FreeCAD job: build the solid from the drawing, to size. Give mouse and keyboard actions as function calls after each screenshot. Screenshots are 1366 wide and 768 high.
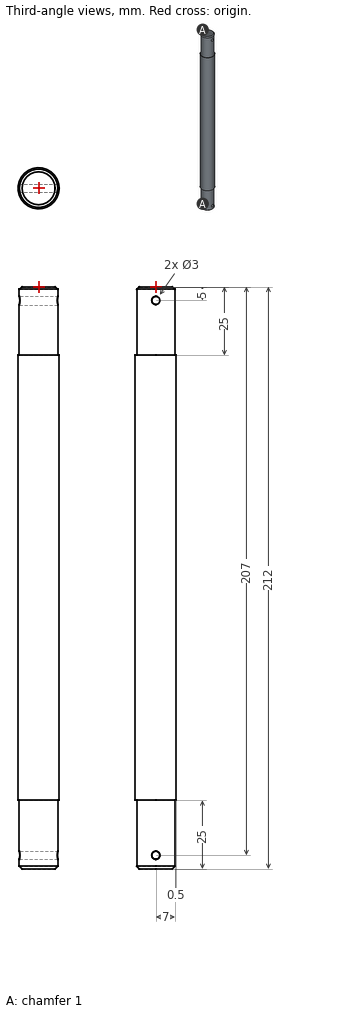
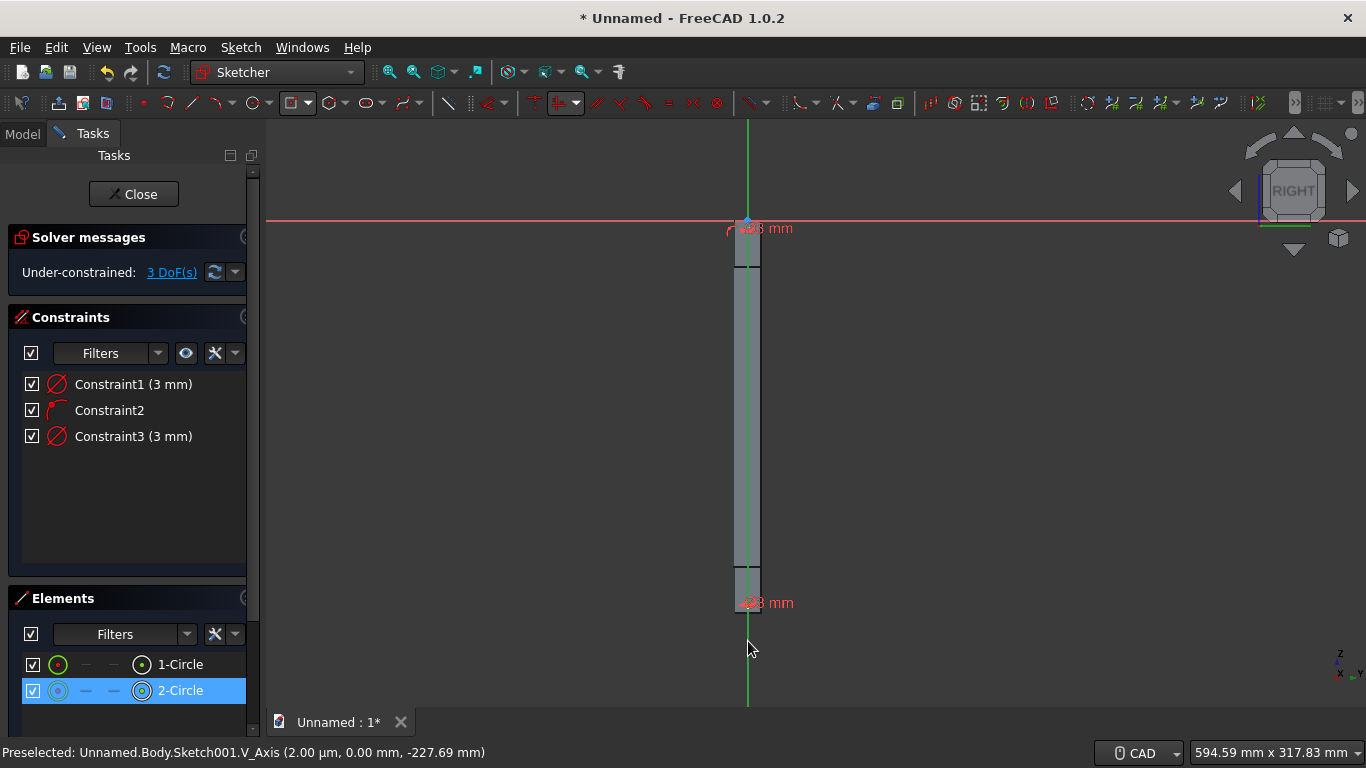
key(c)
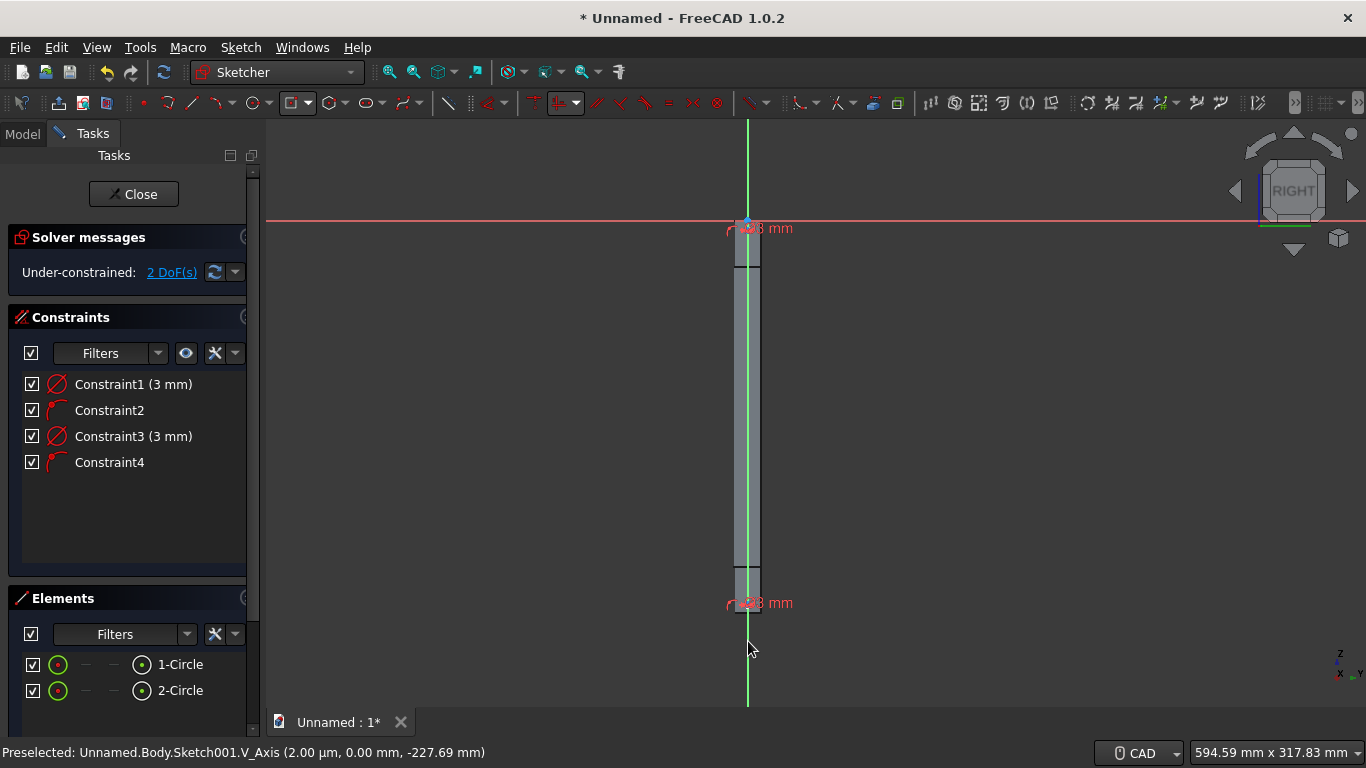
scroll(748, 230, up, 8)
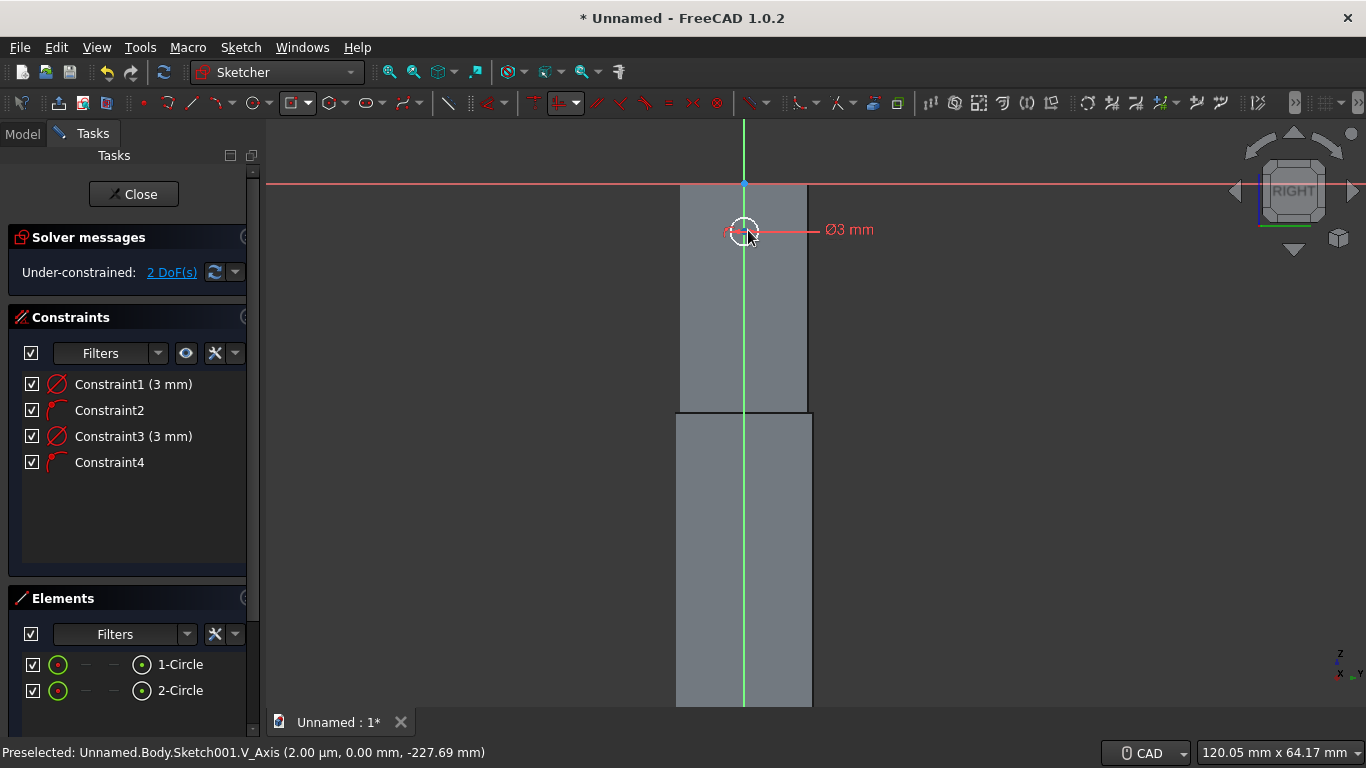
click(744, 232)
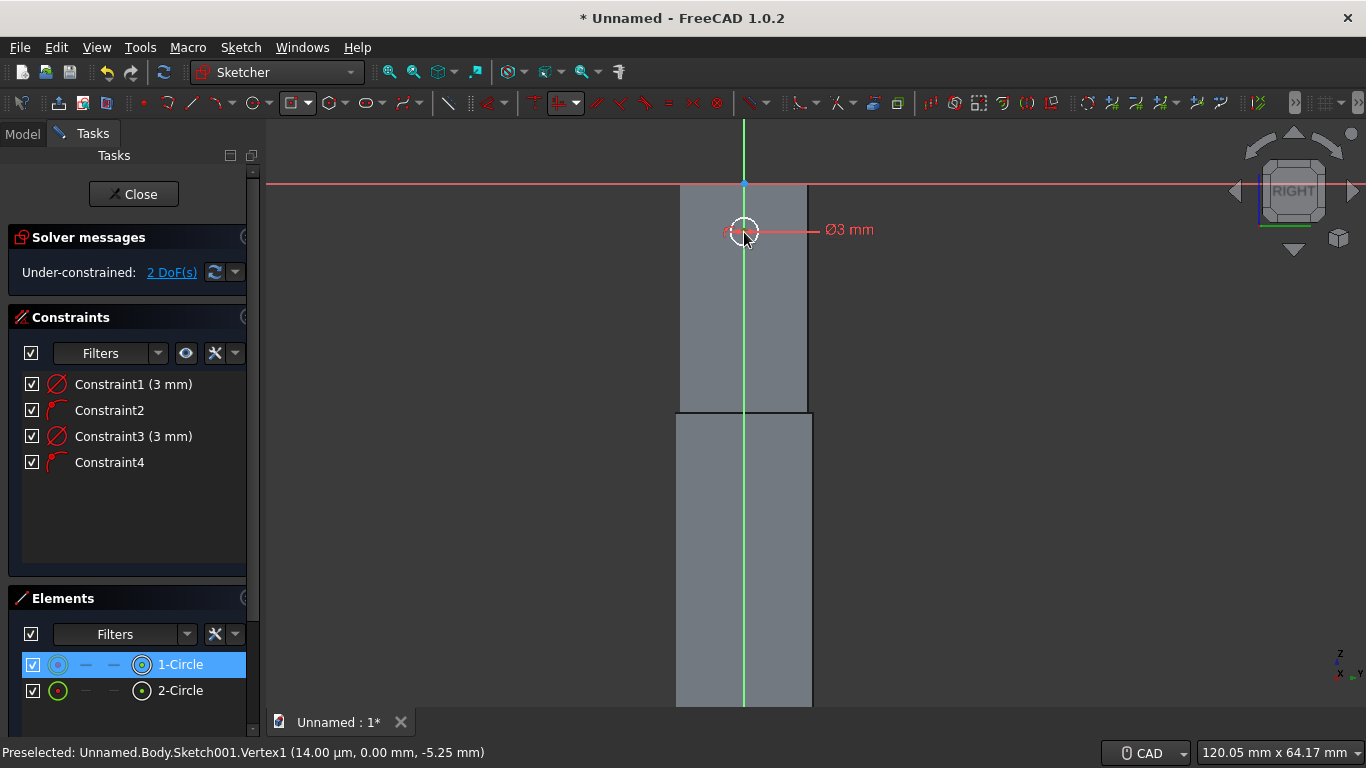
click(506, 104)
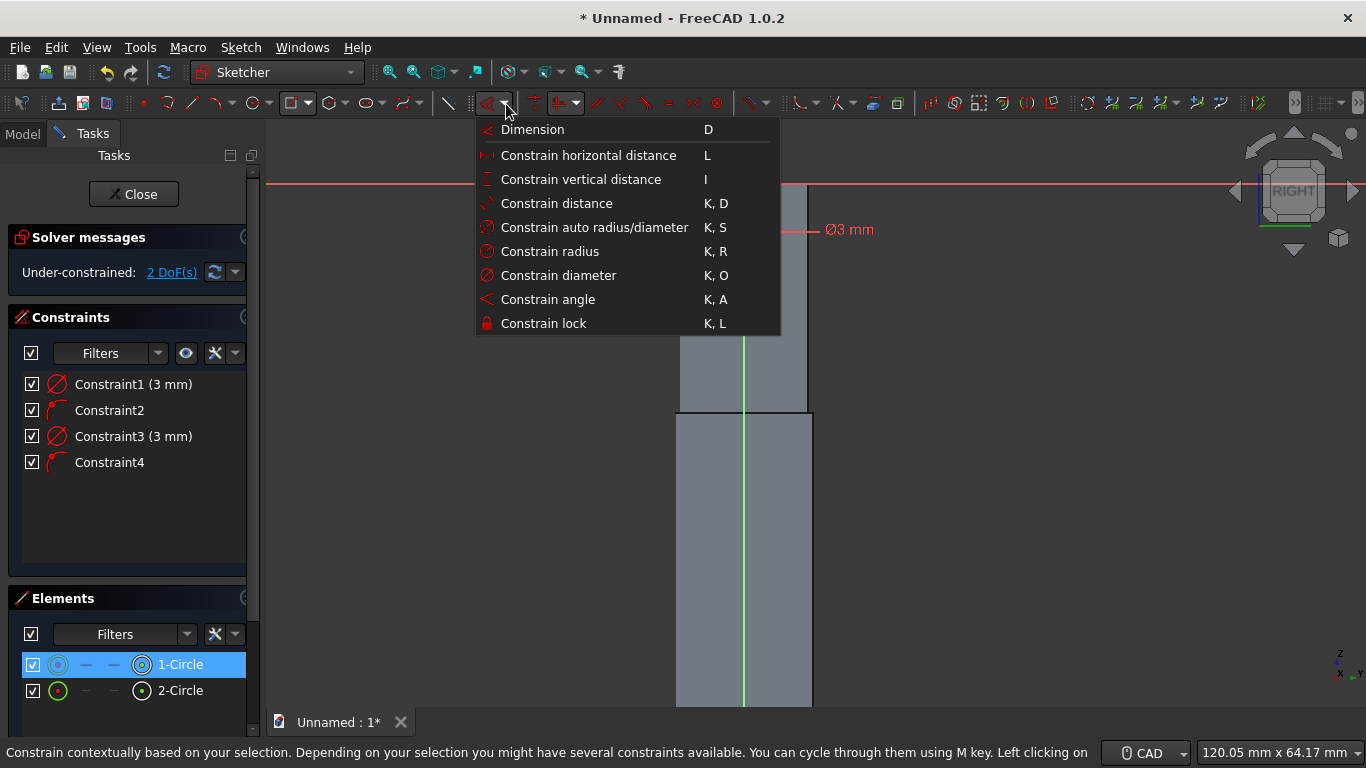
click(628, 179)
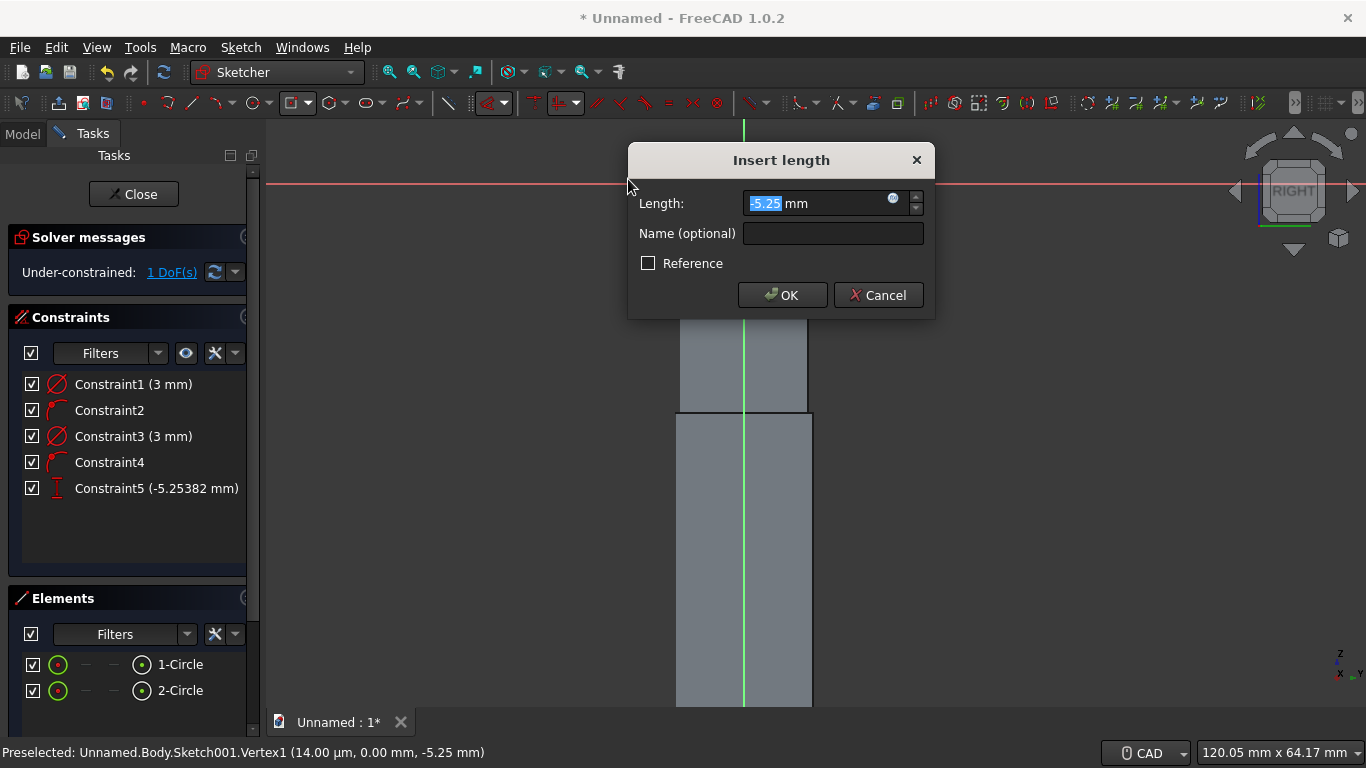
text(-5)
key(Return)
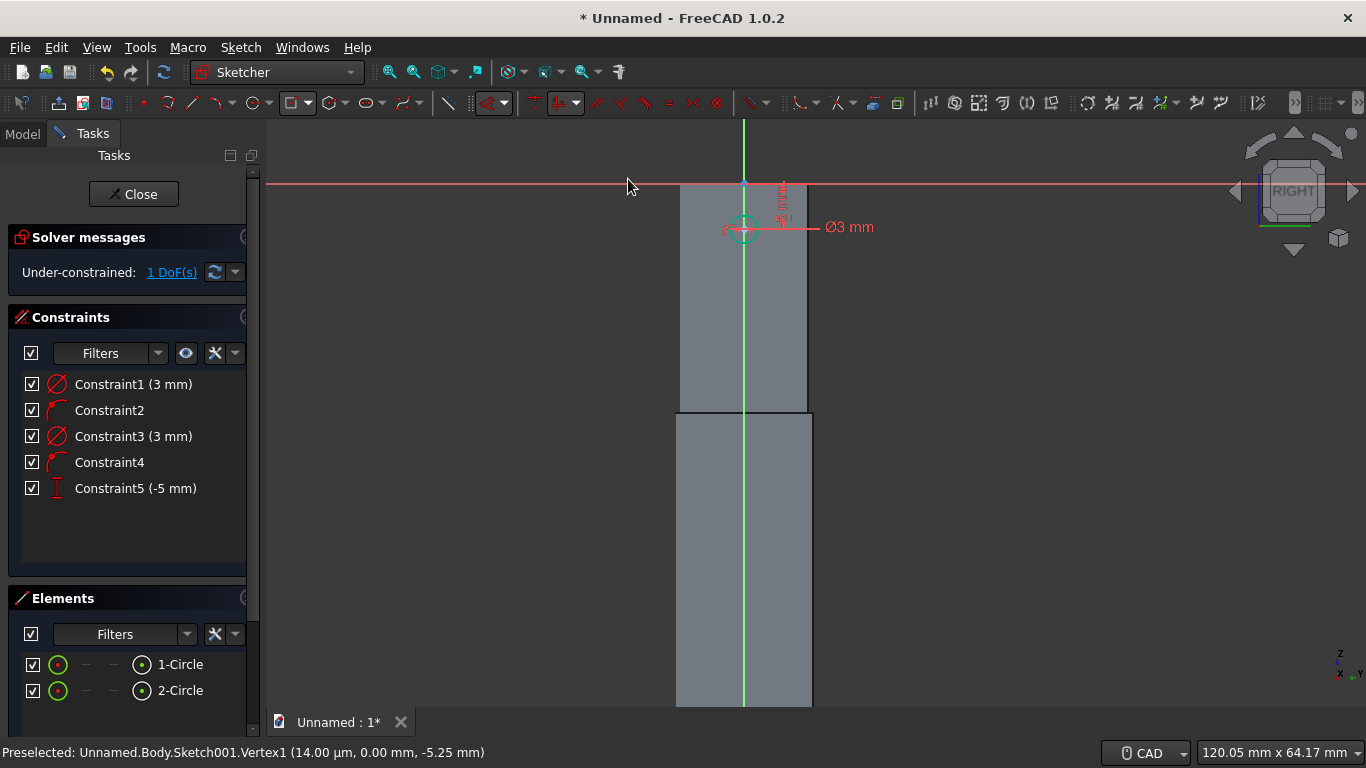
scroll(748, 229, down, 8)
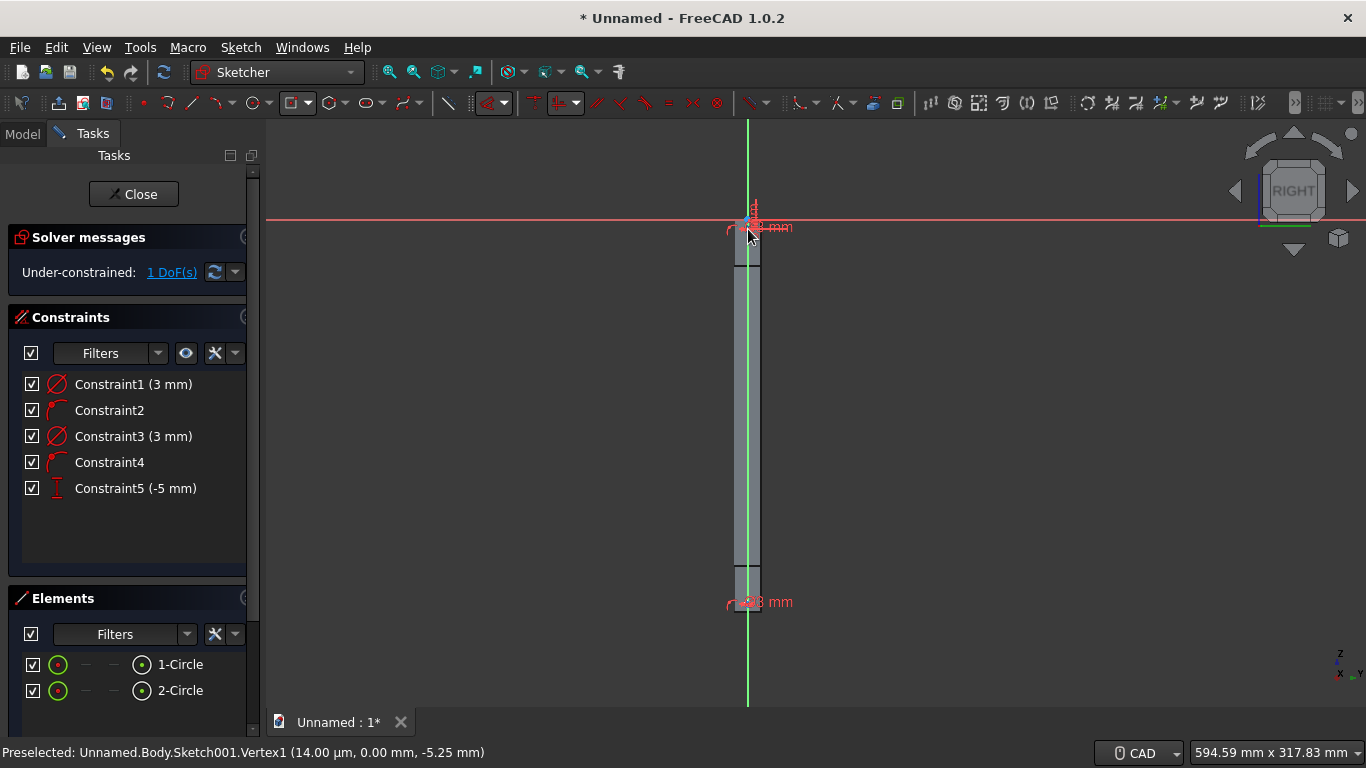
click(748, 604)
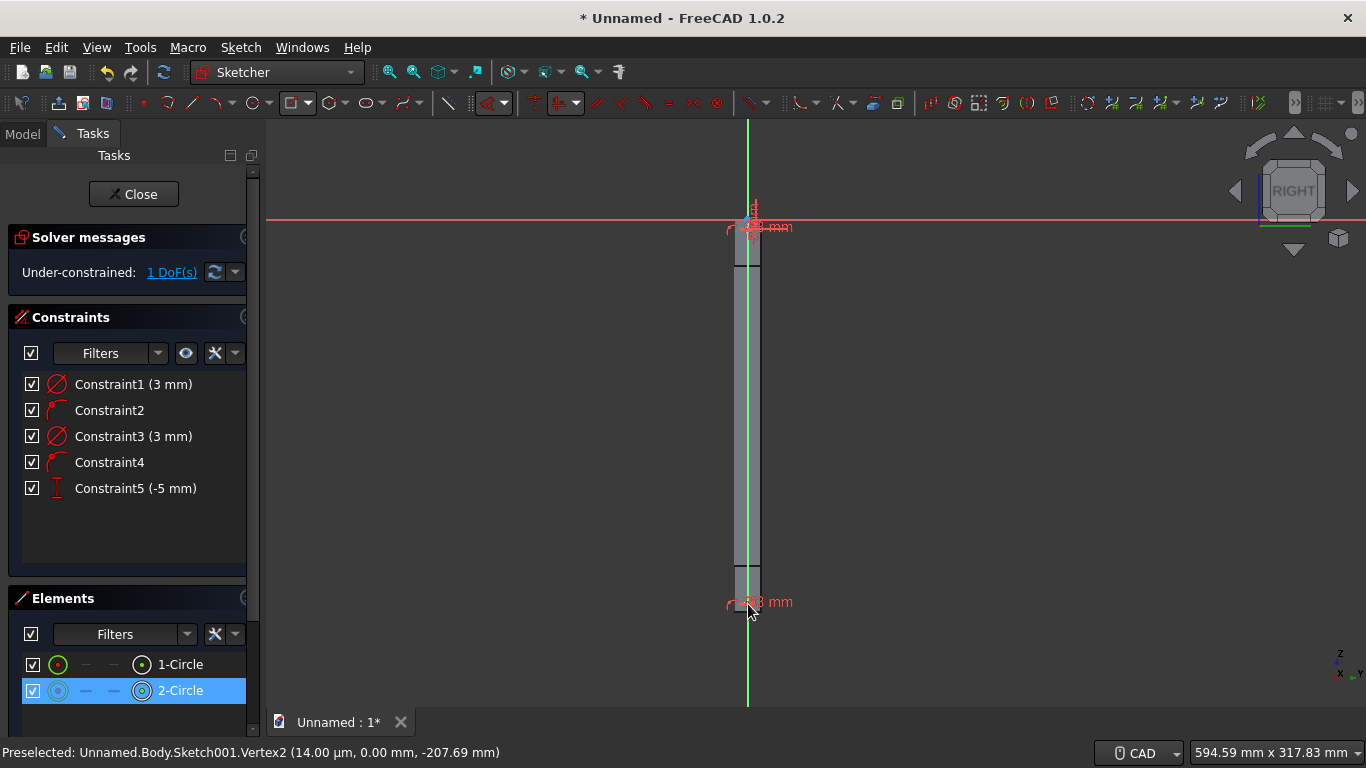
click(506, 104)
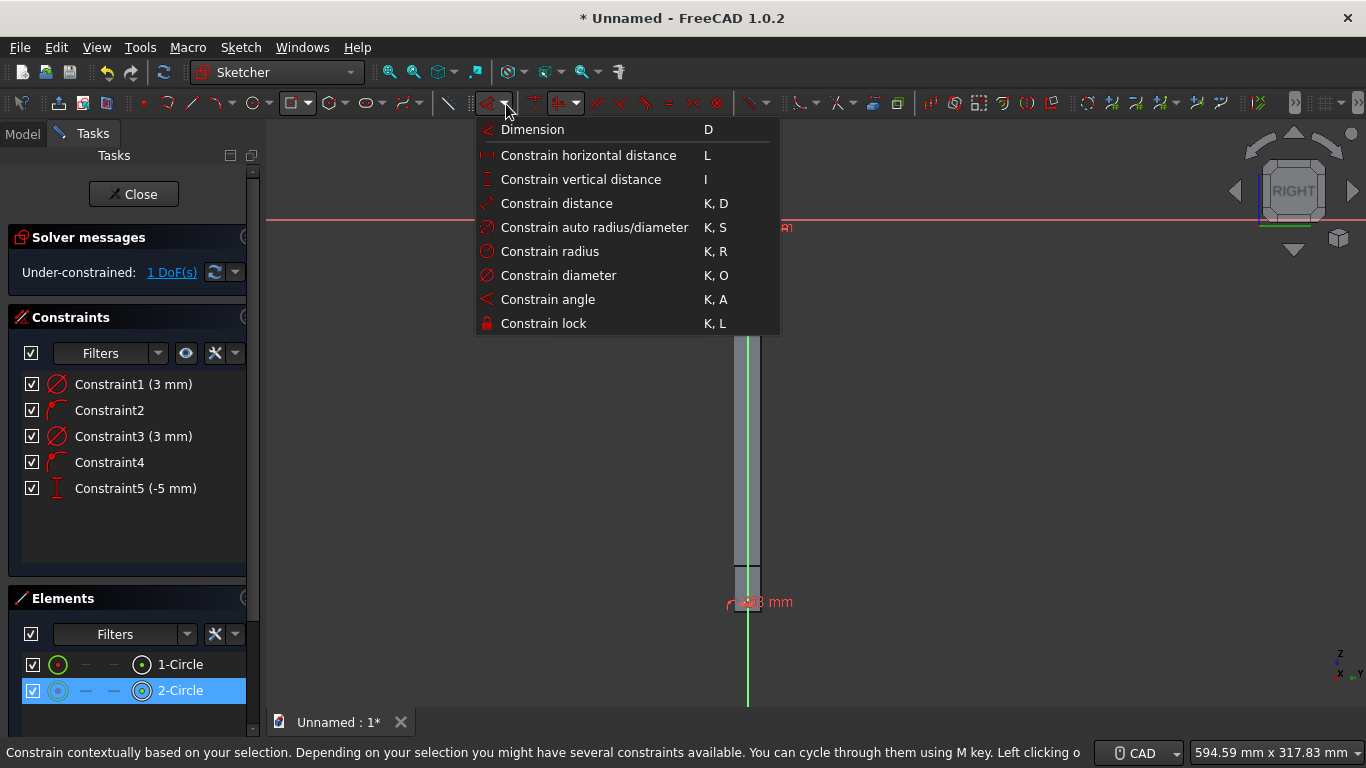
click(628, 179)